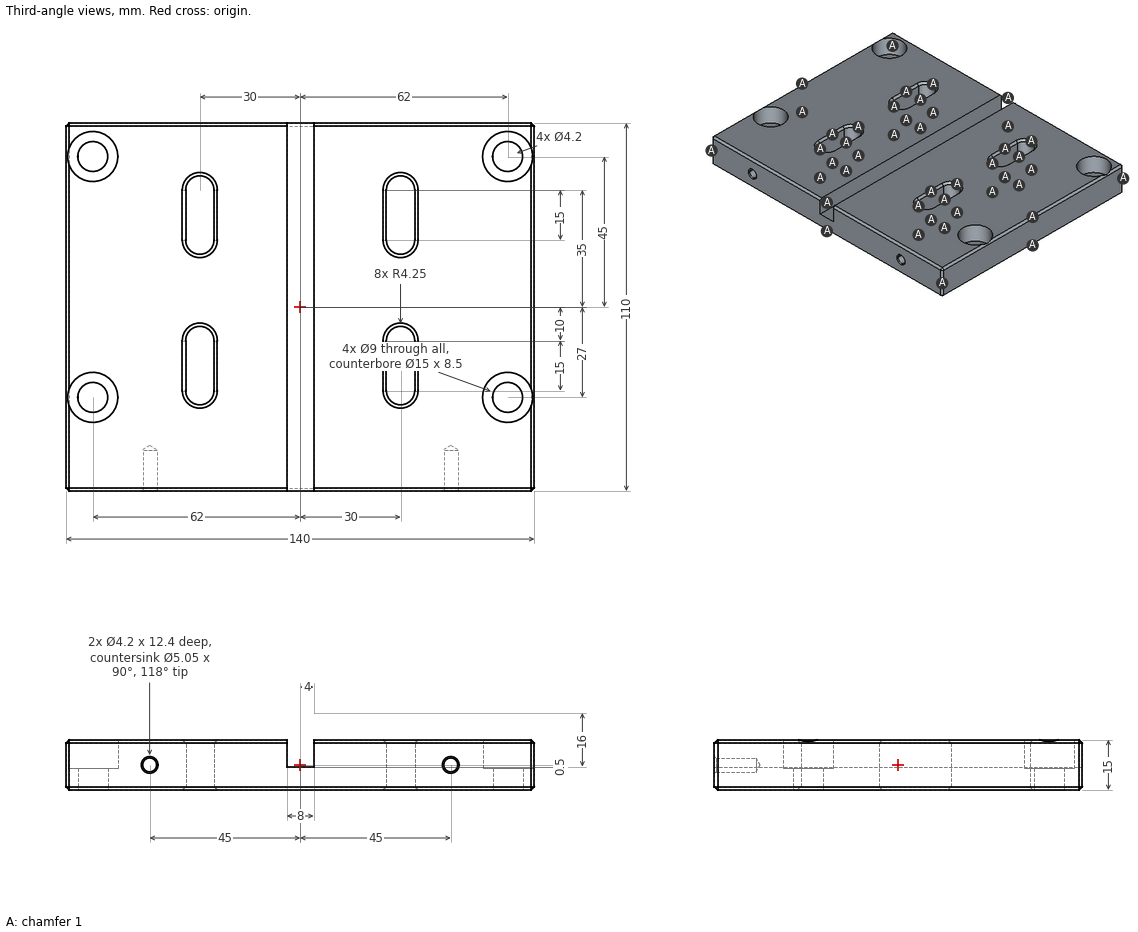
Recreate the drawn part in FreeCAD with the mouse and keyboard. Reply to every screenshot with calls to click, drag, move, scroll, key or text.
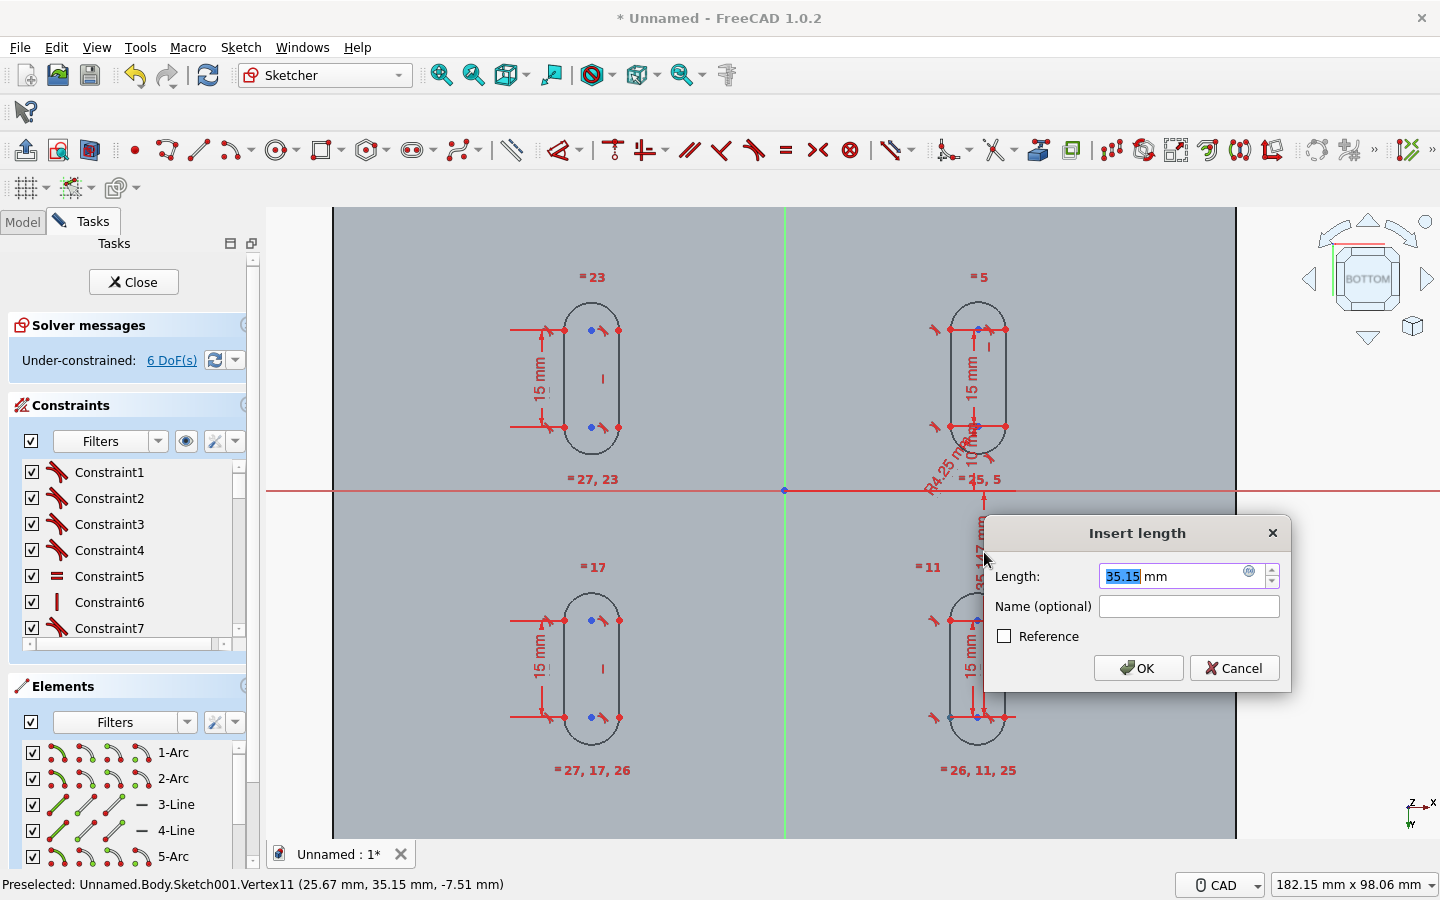
text(35)
key(Return)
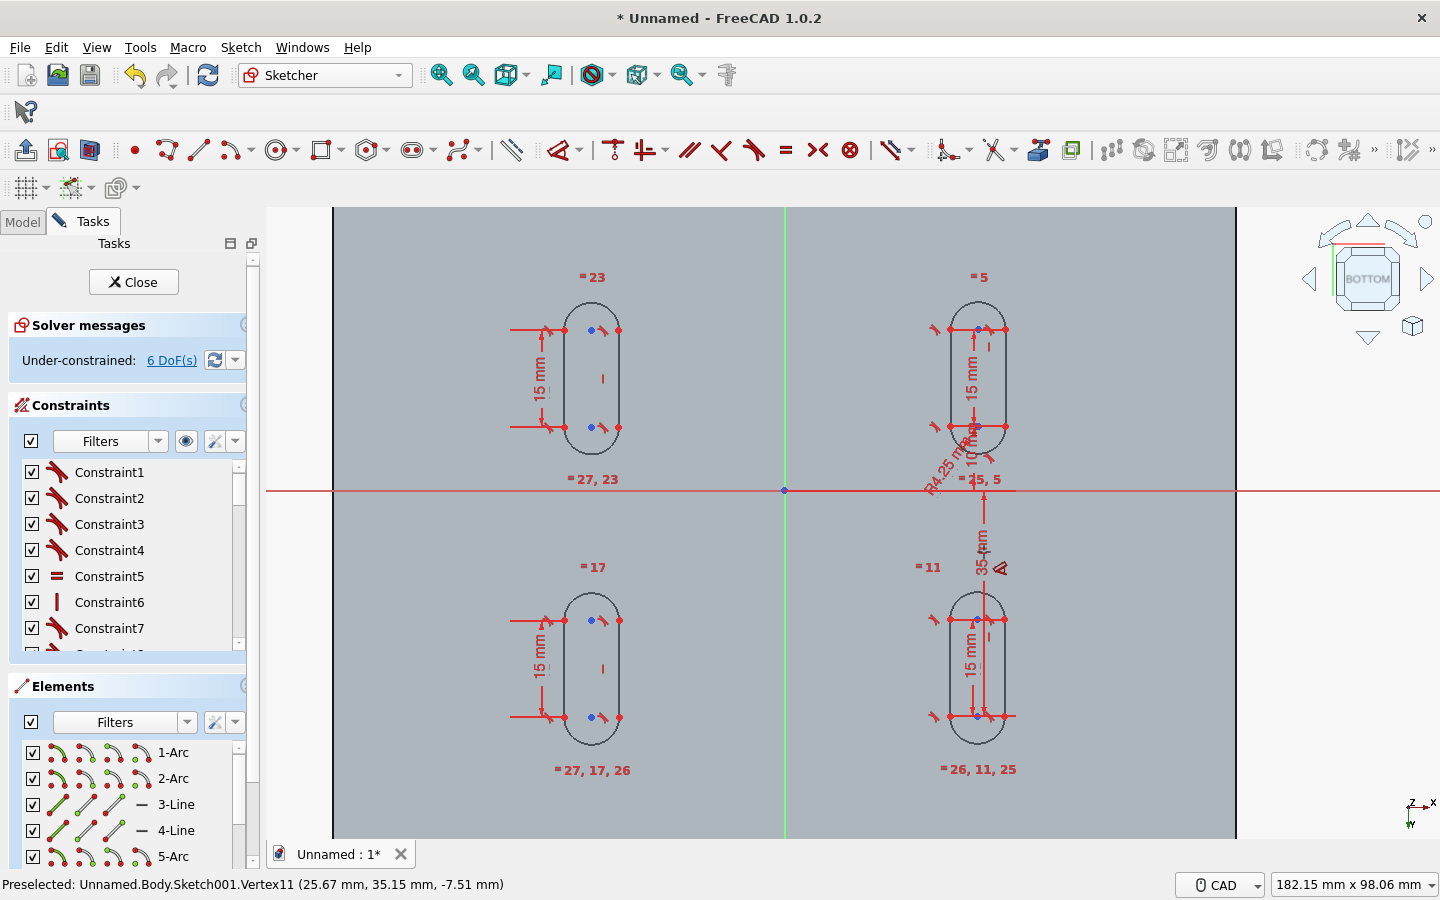
click(564, 717)
click(530, 604)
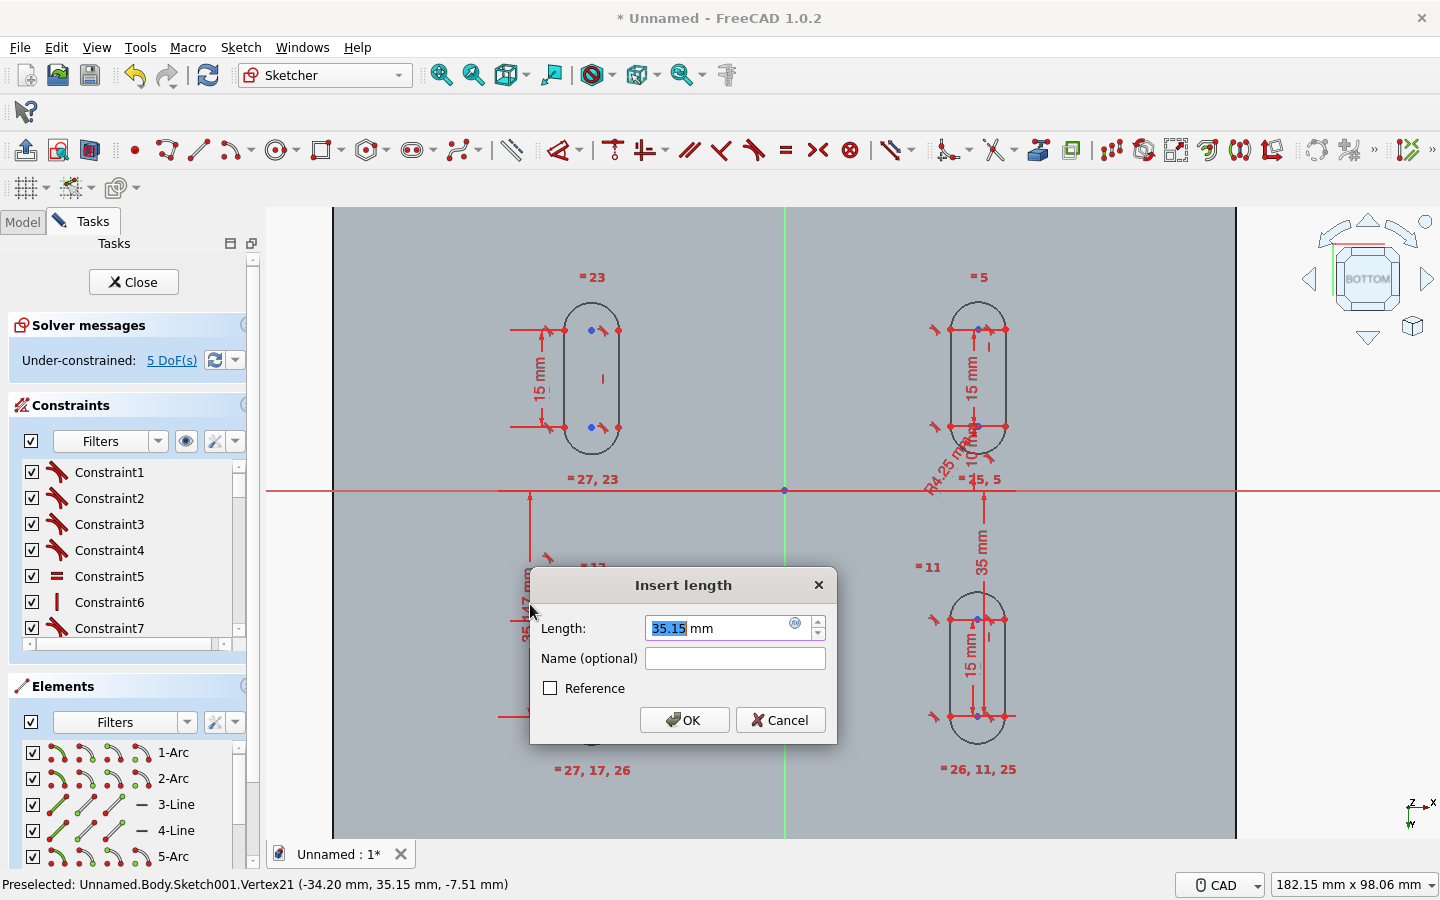
text(35)
key(Return)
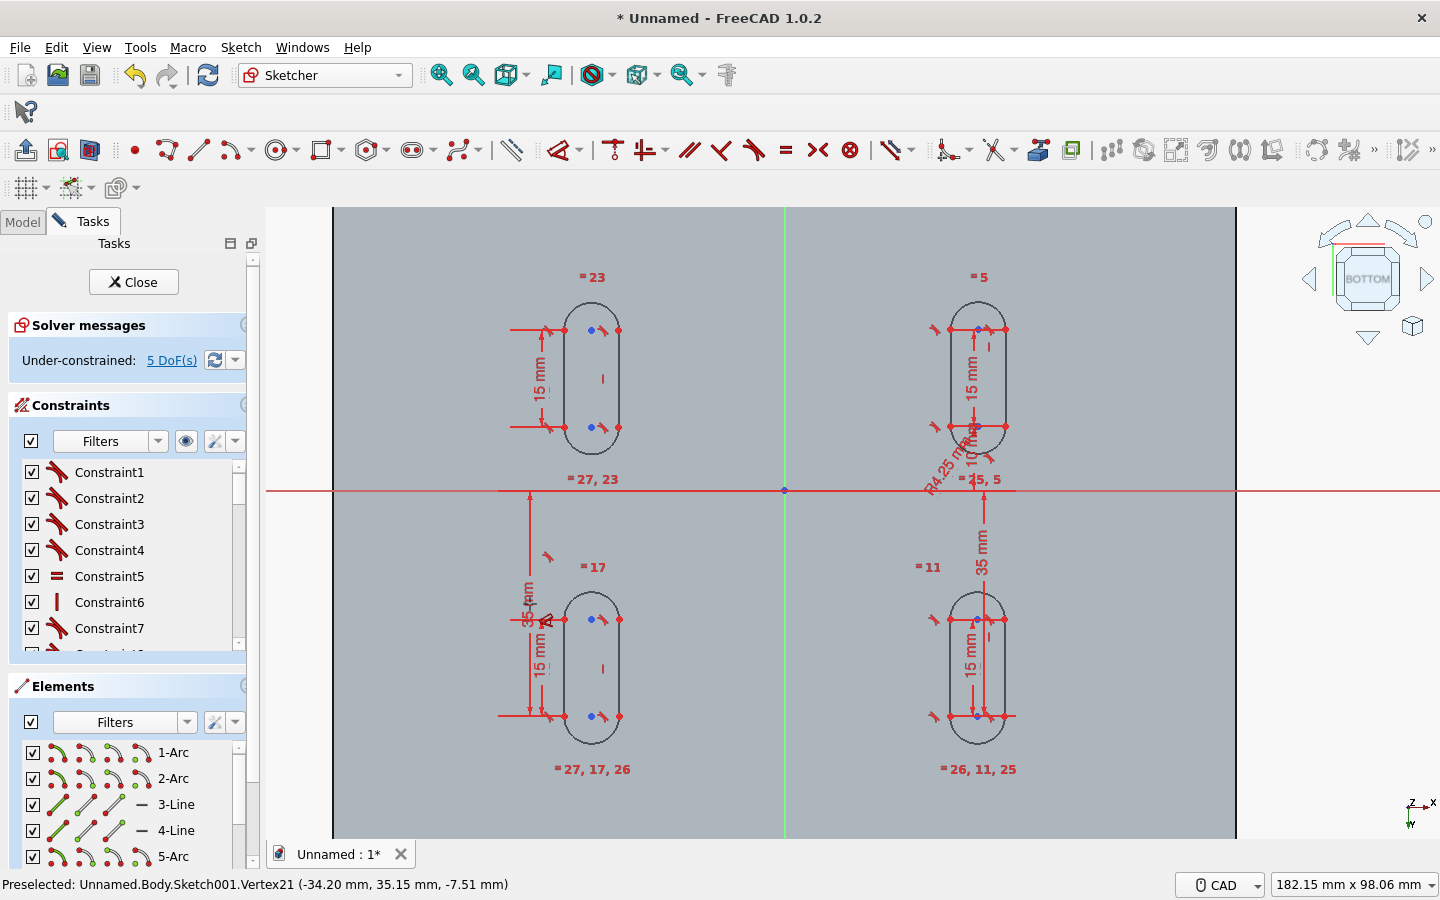
click(564, 427)
click(530, 459)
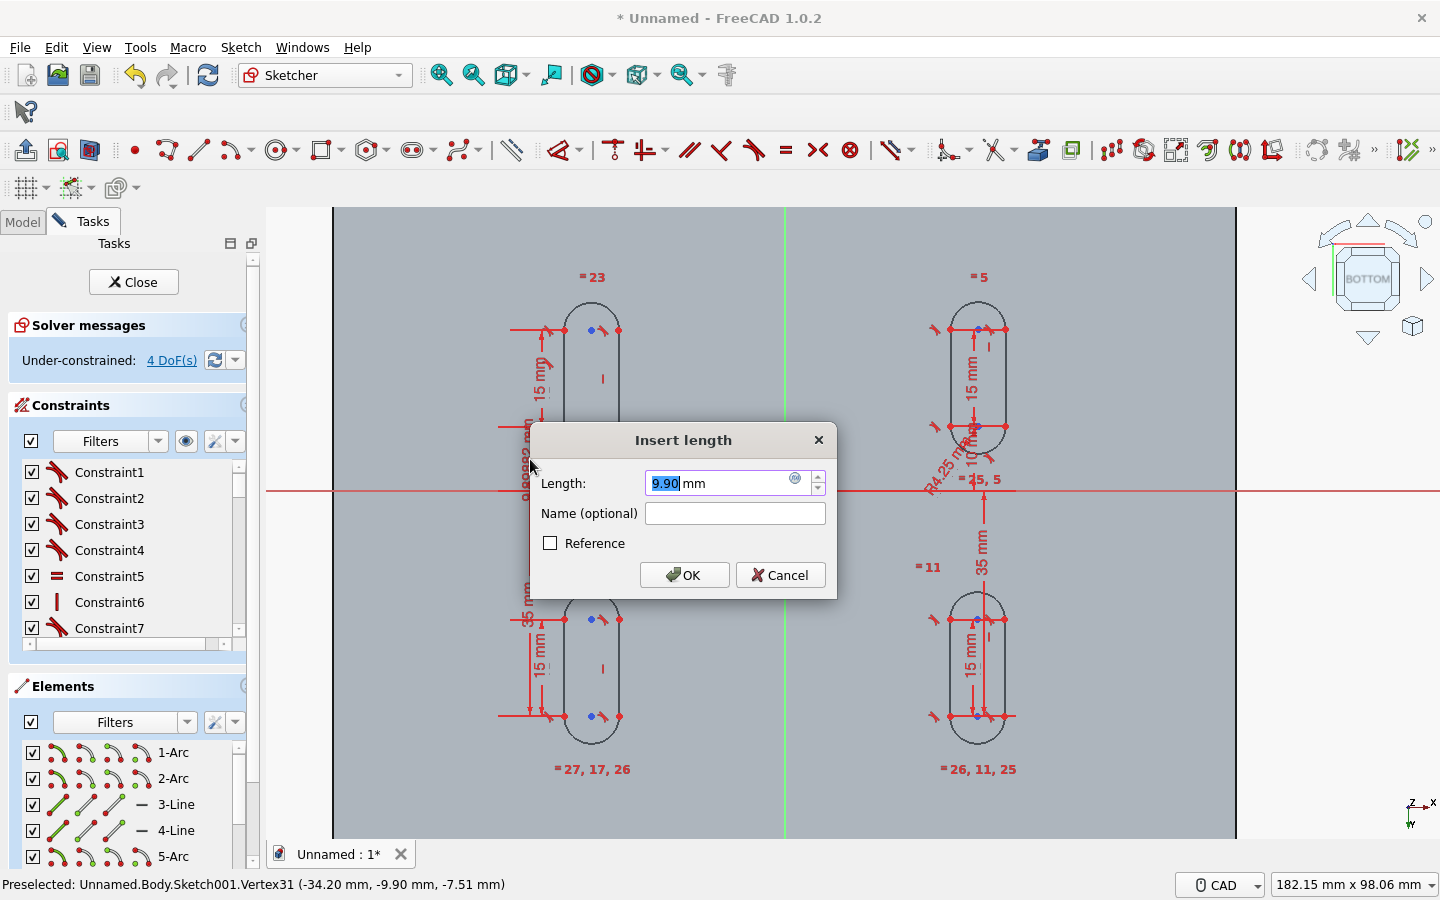
text(10)
key(Return)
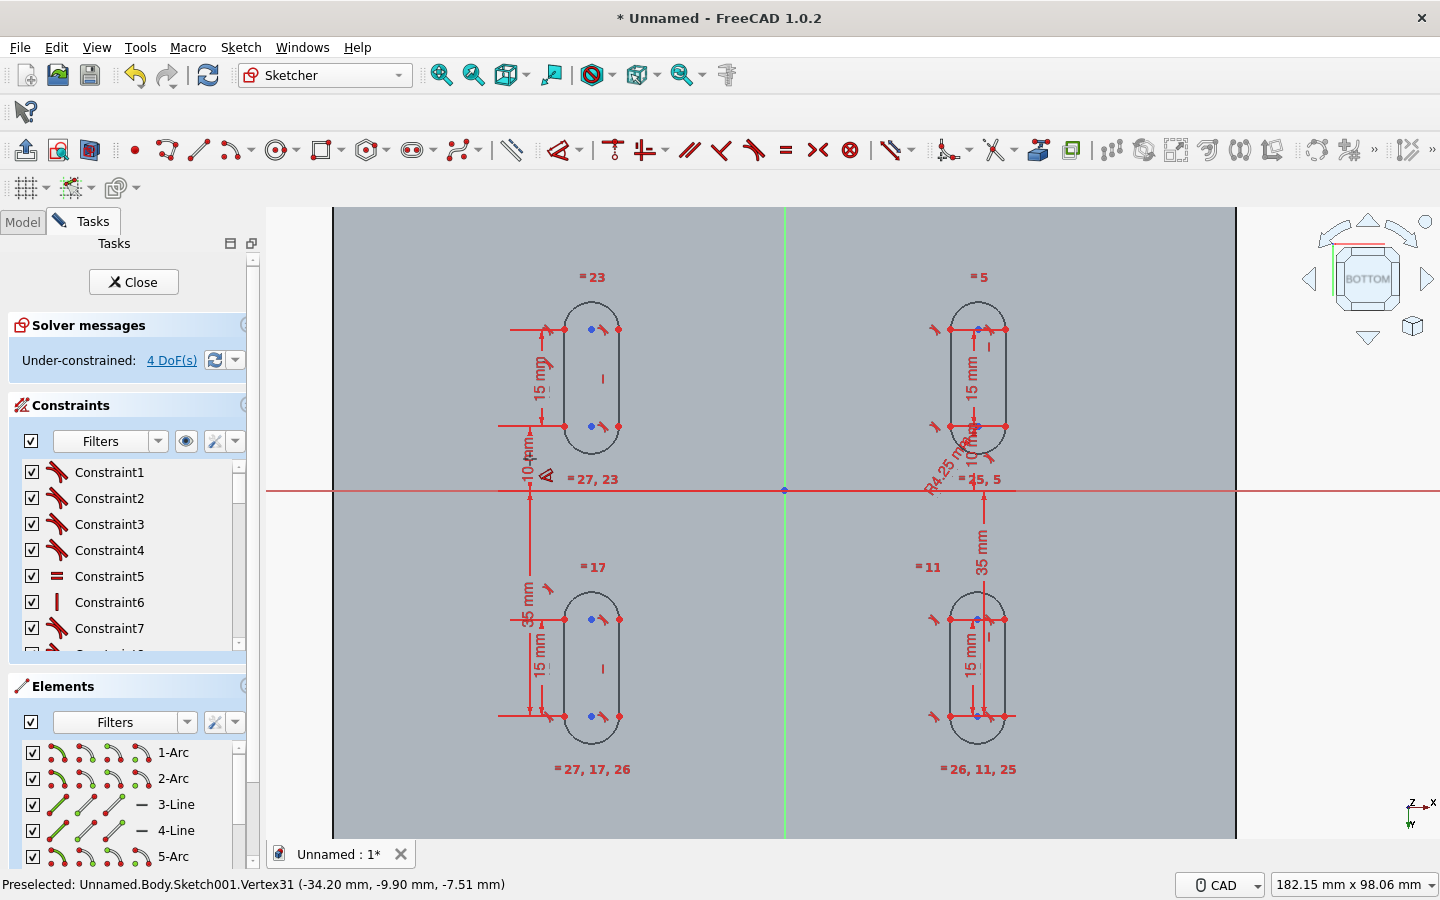
click(978, 426)
click(881, 392)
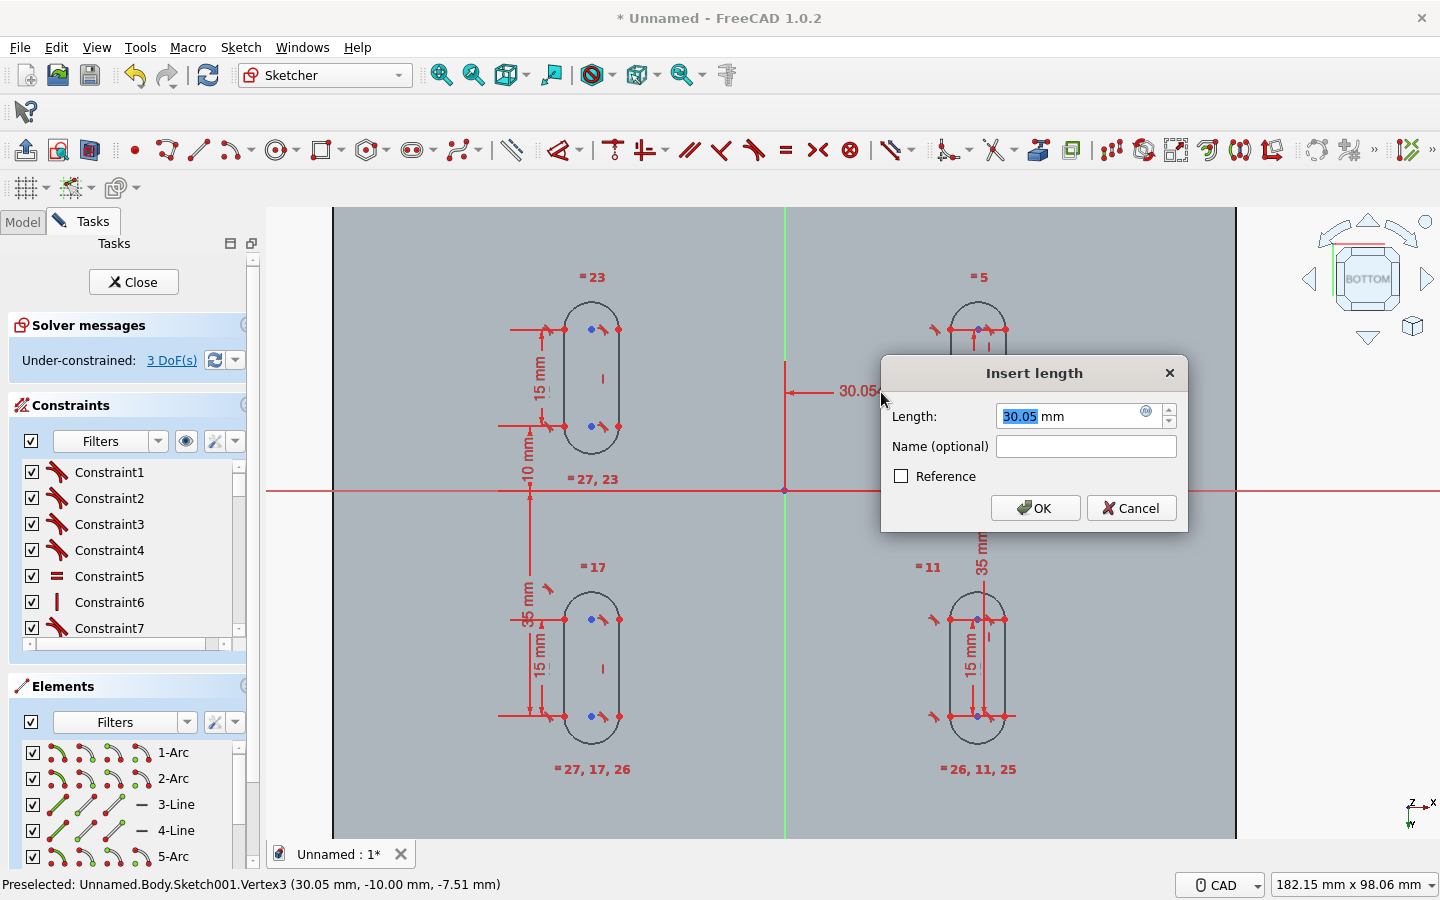
text(30)
key(Return)